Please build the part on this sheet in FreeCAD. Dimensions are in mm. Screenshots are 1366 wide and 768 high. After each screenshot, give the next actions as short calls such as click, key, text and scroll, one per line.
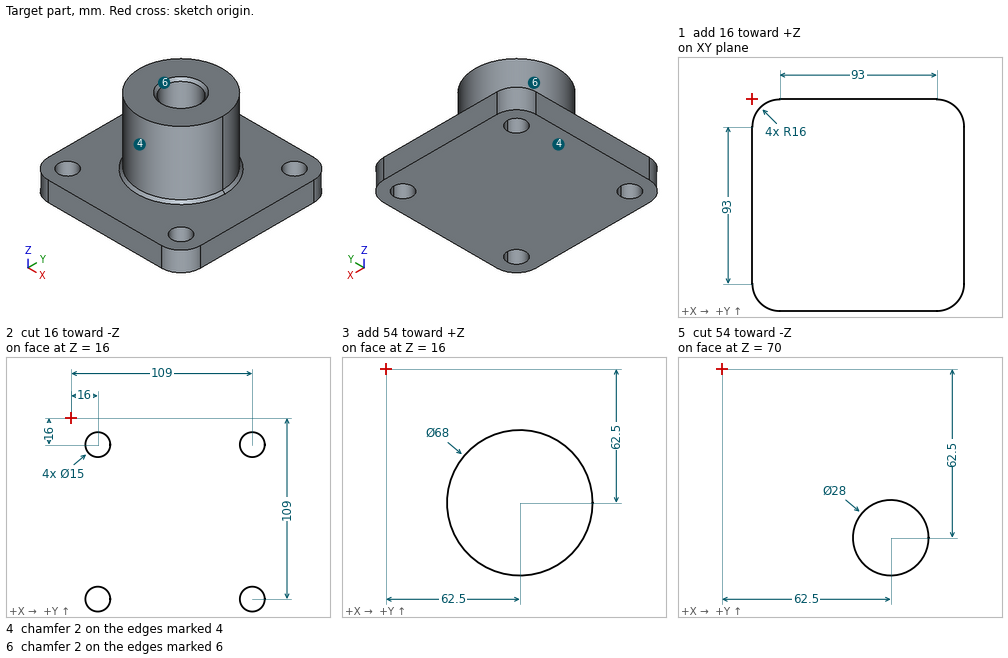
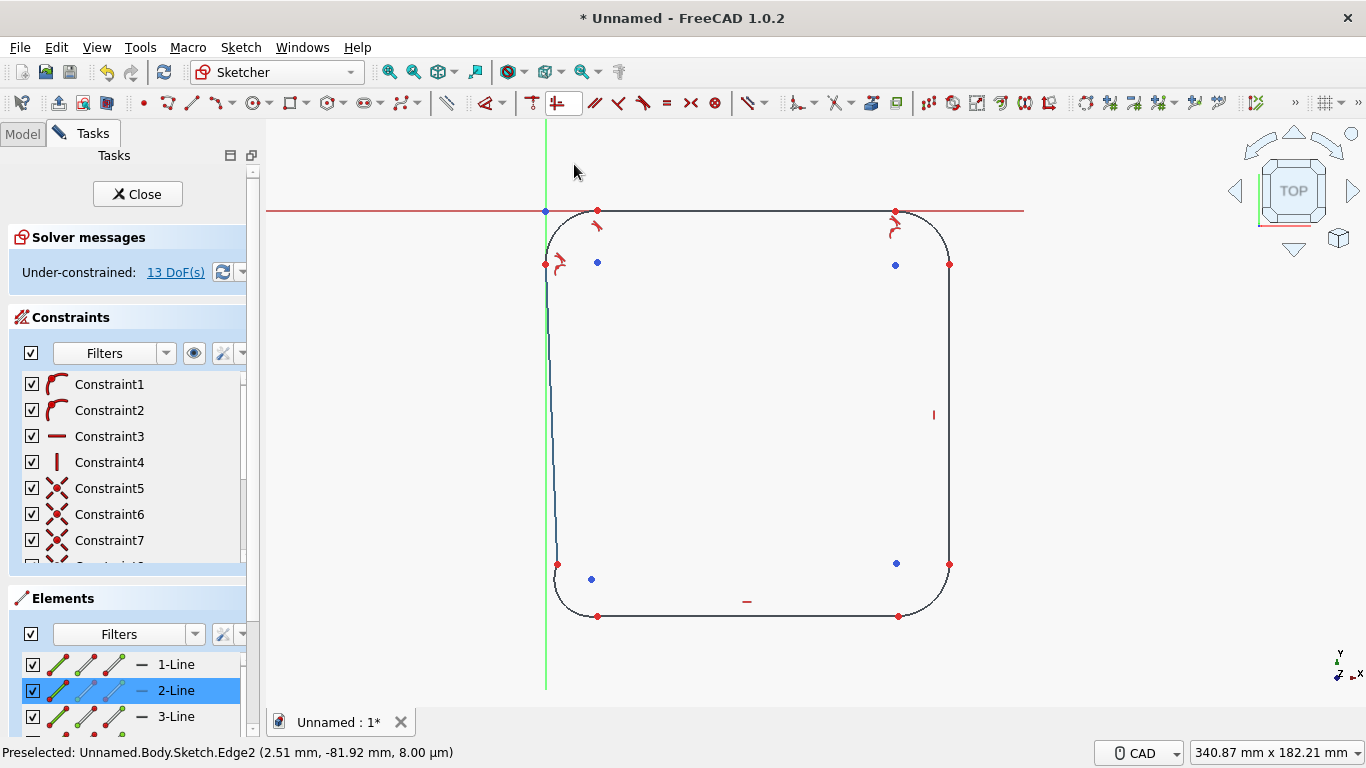
scroll(555, 588, up, 2)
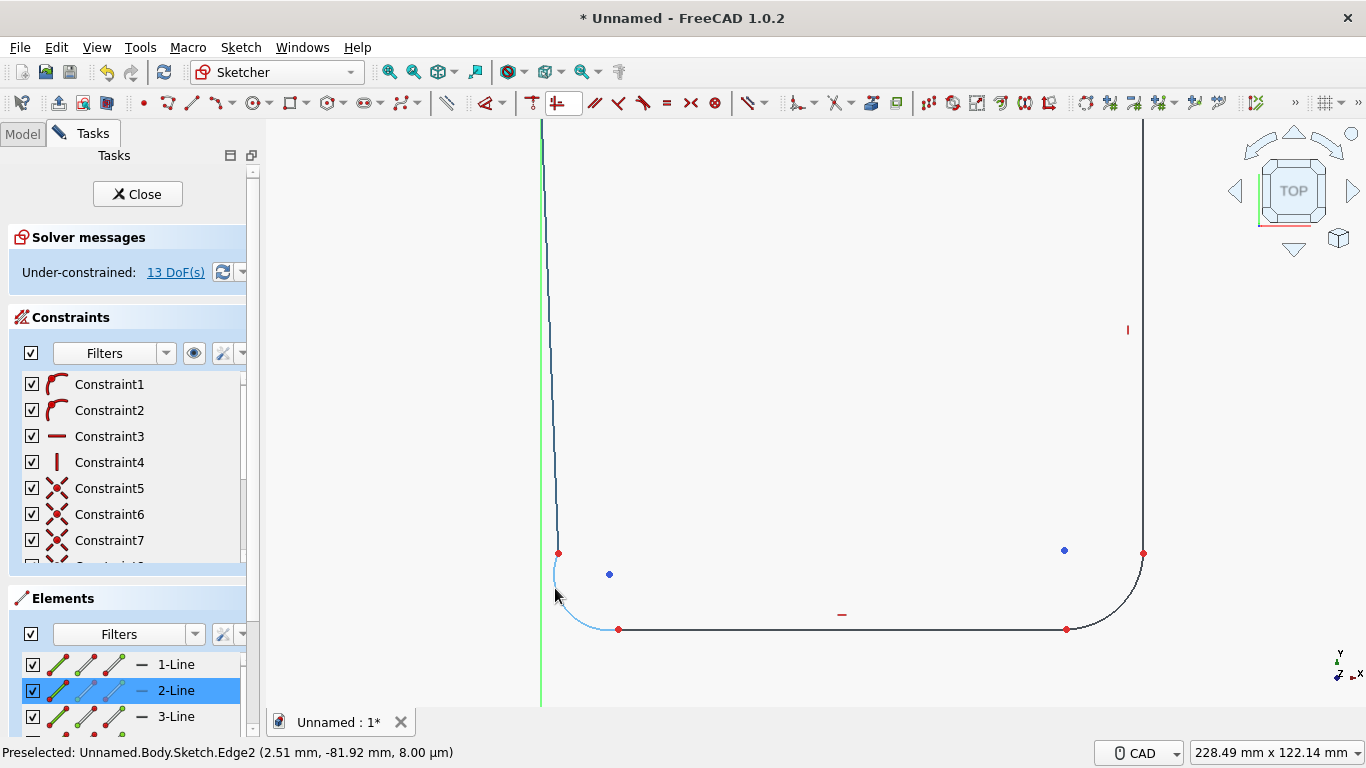
click(556, 588)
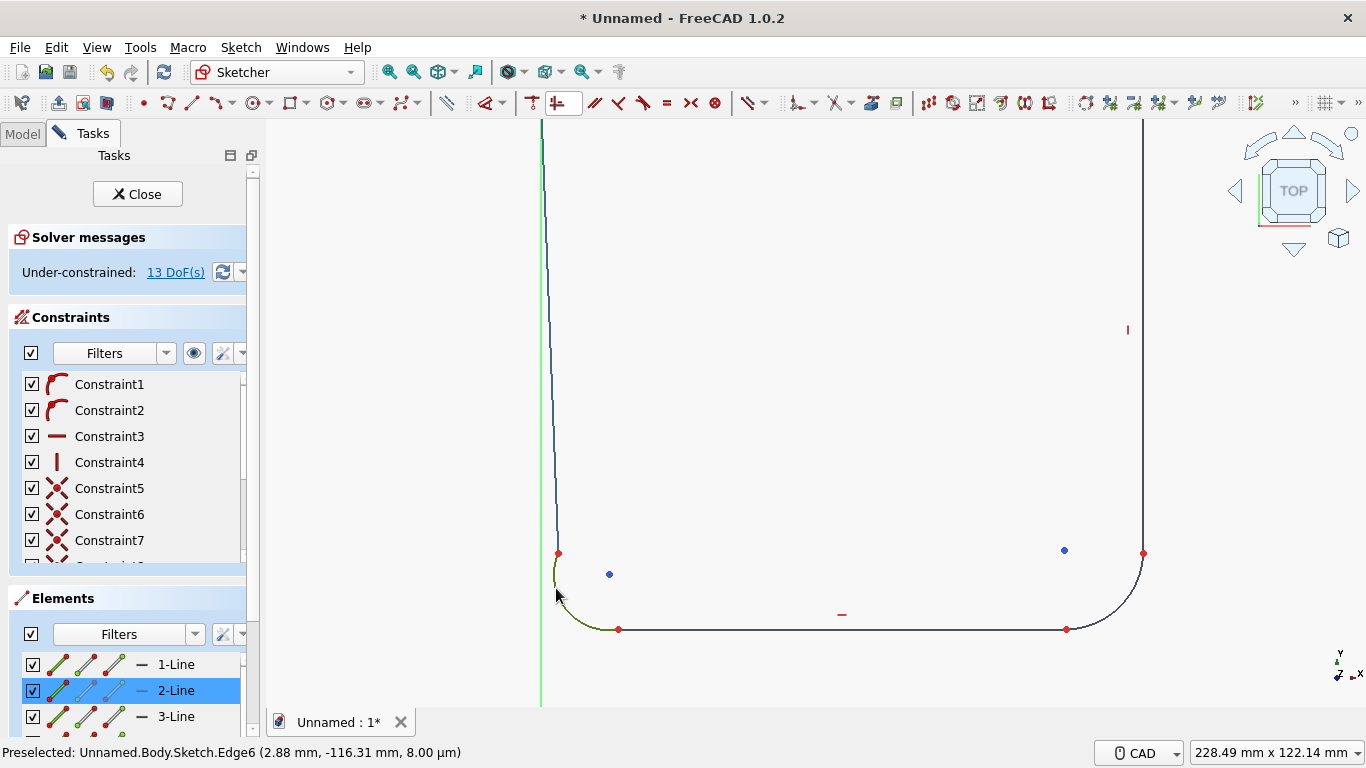
key(t)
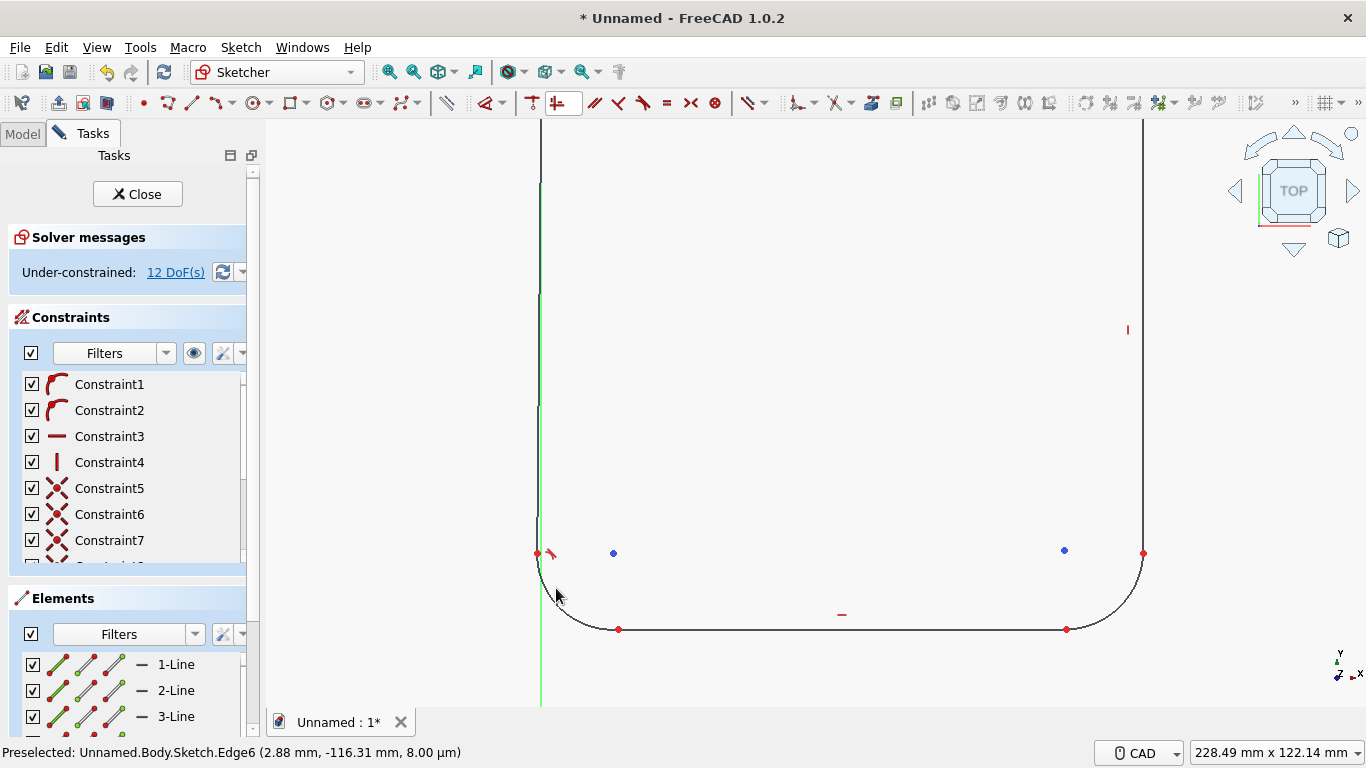
click(753, 630)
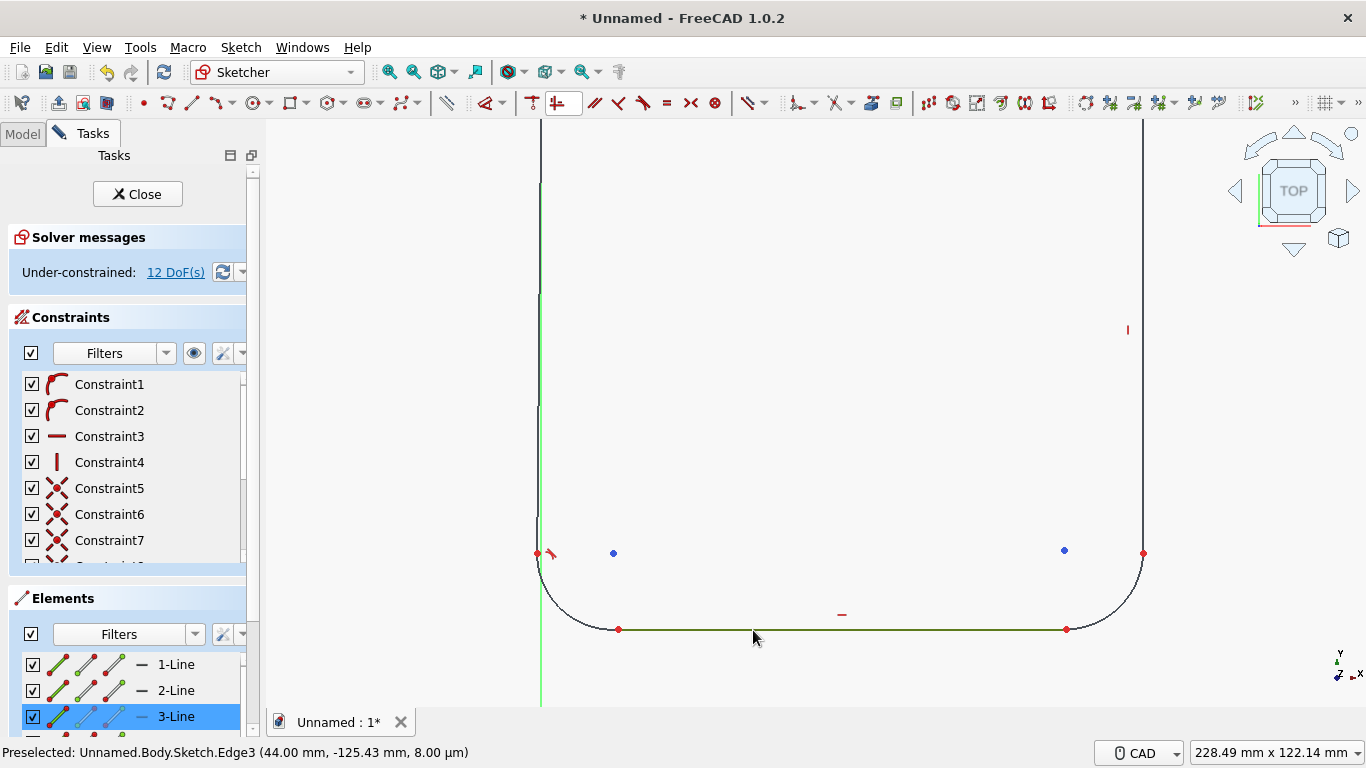
click(582, 623)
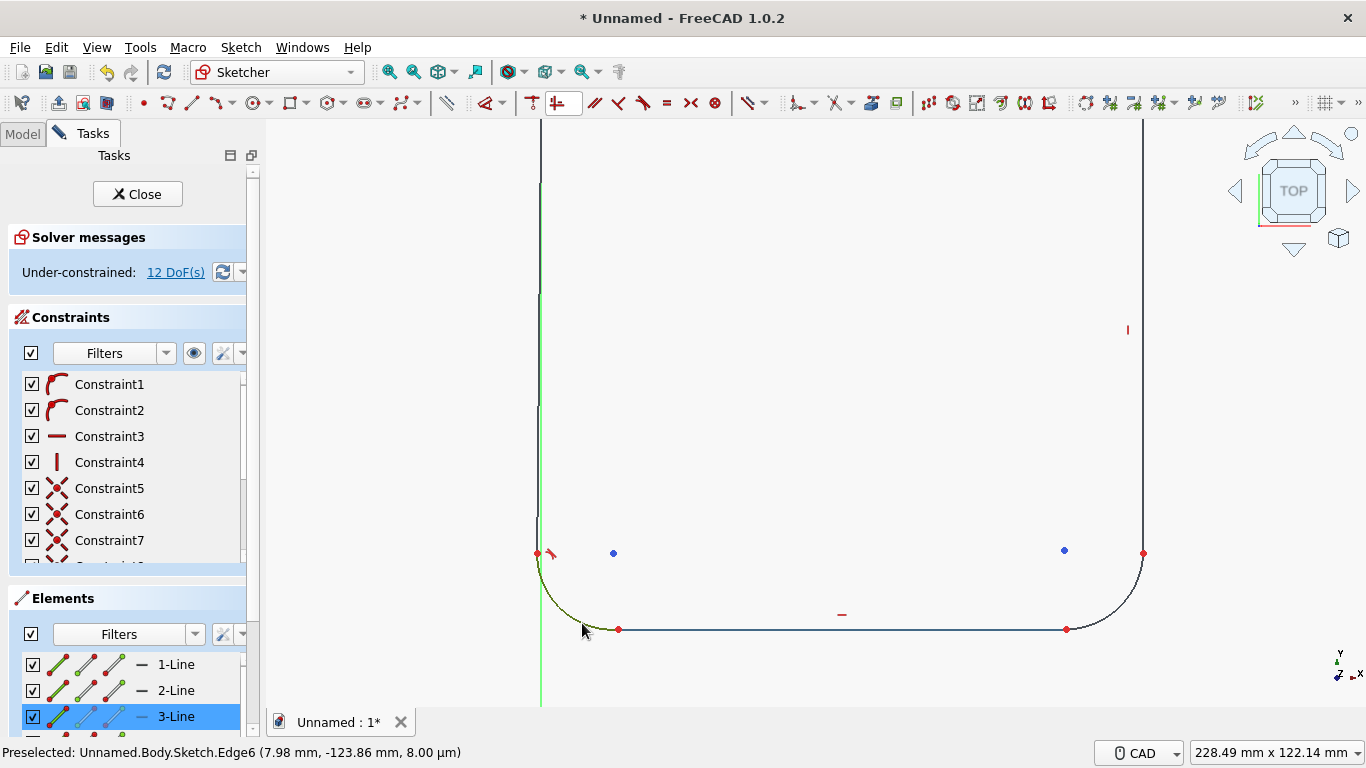
key(t)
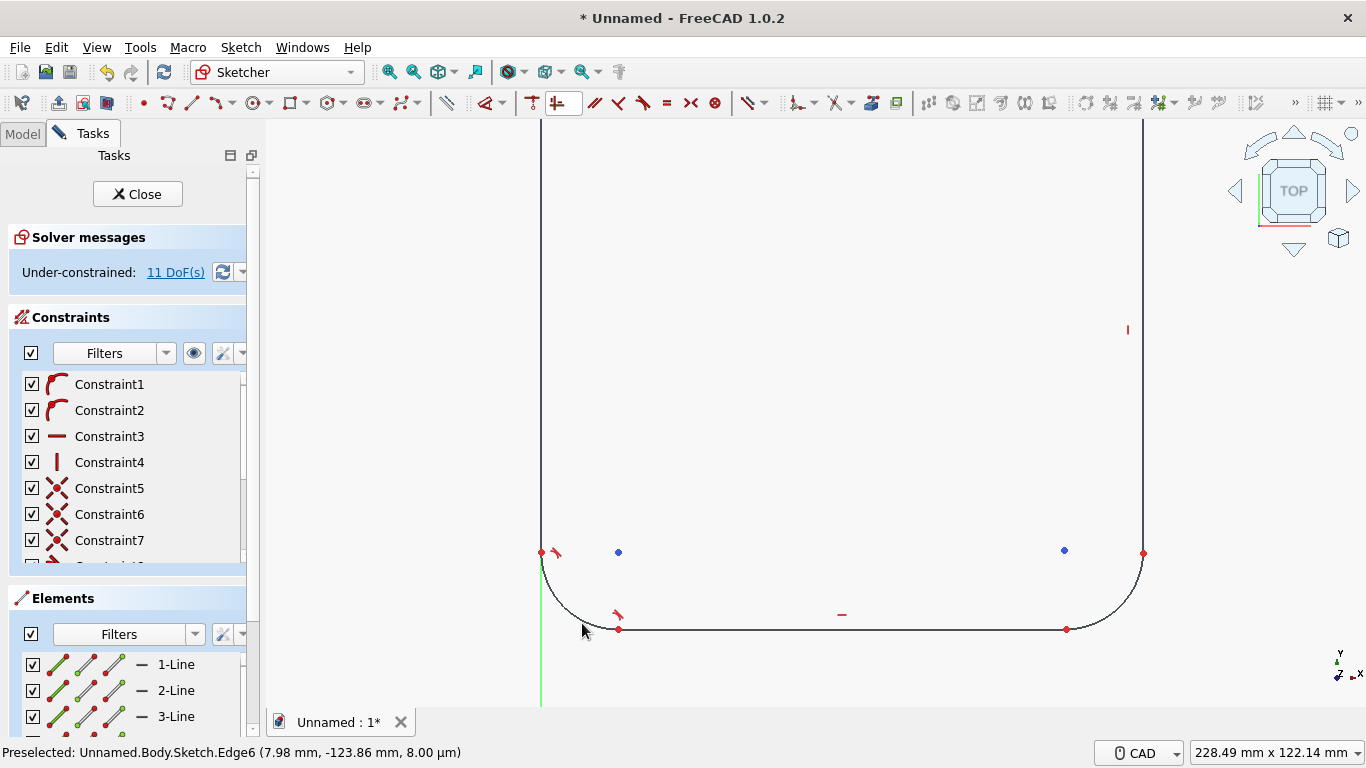
click(753, 630)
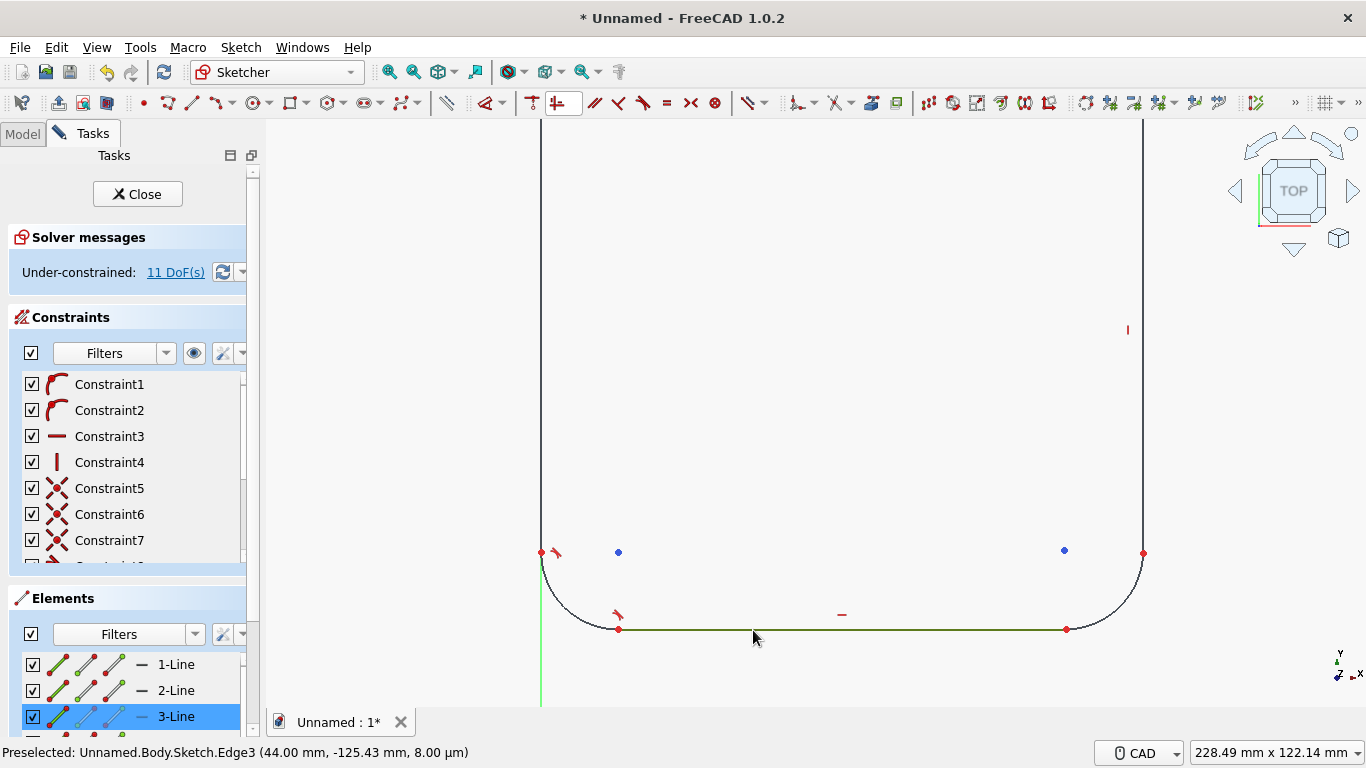
click(1101, 621)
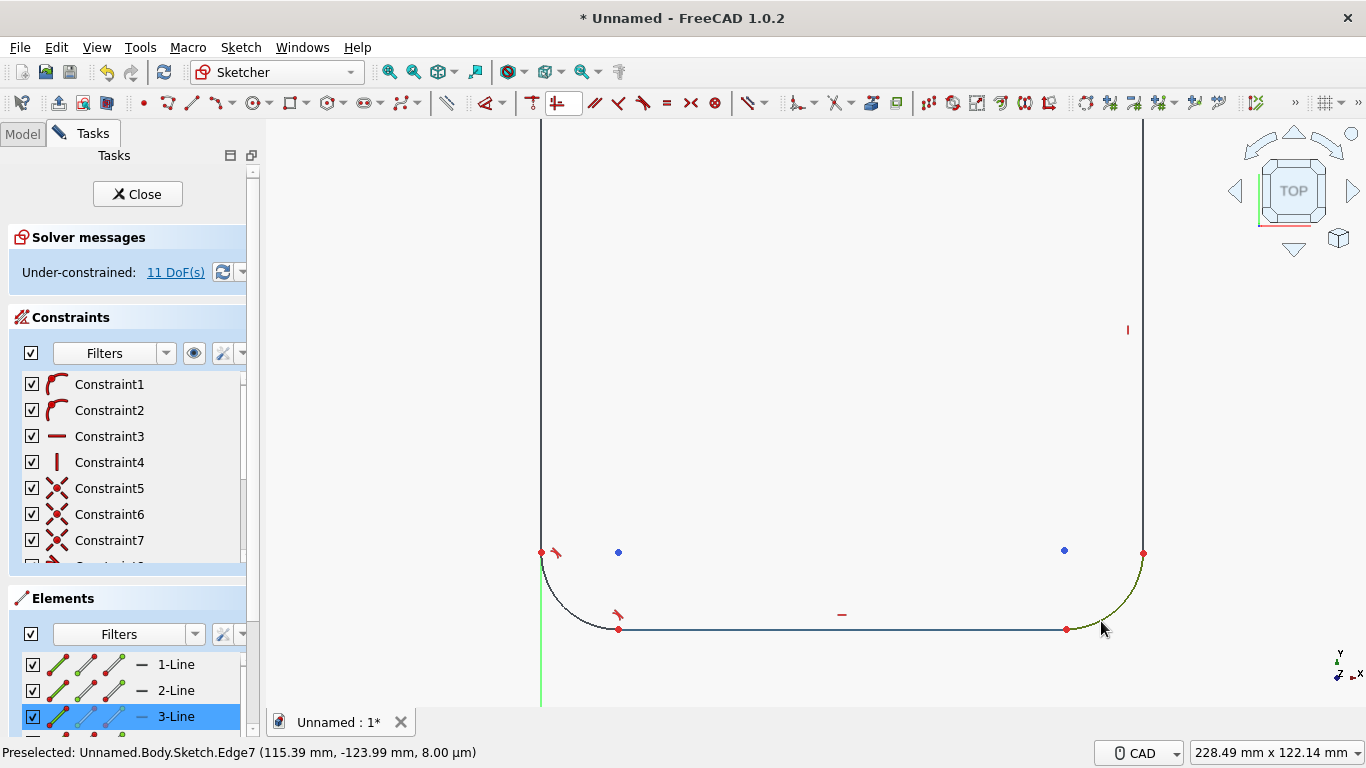
key(t)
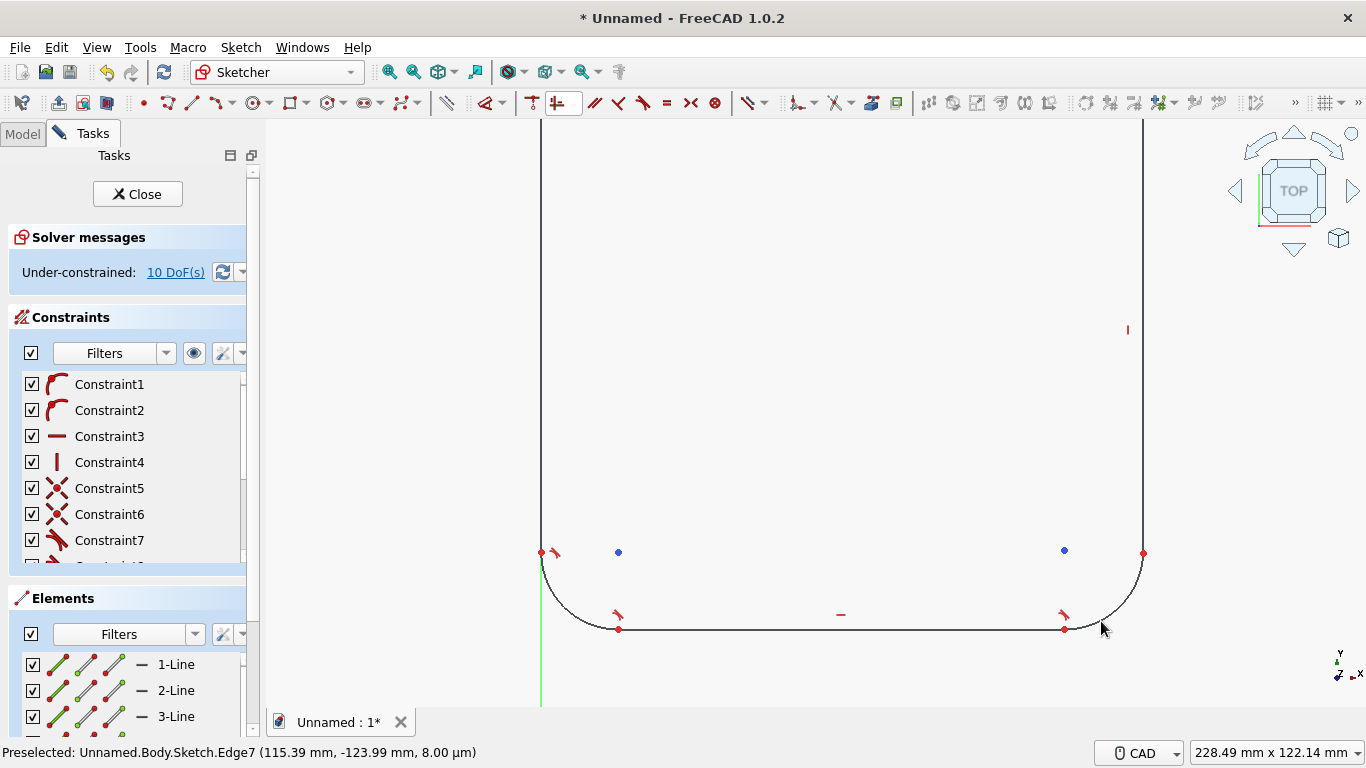
click(1143, 419)